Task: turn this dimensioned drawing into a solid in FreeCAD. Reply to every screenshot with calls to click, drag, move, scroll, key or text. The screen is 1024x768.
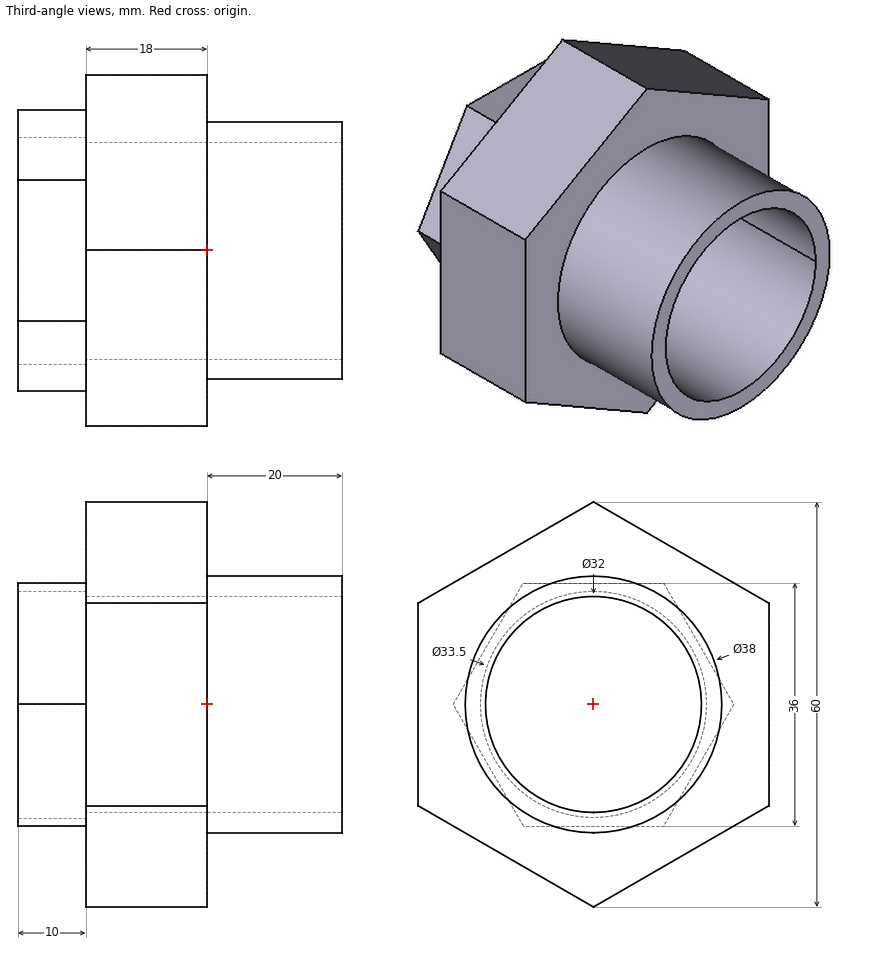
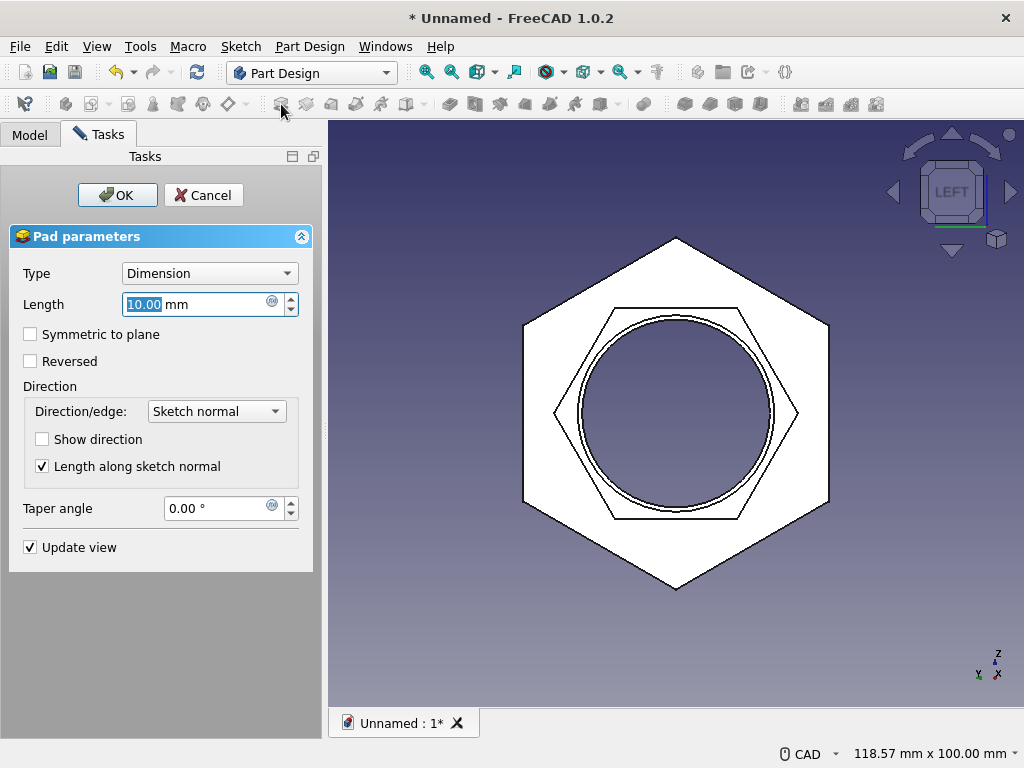
text(10)
key(Tab)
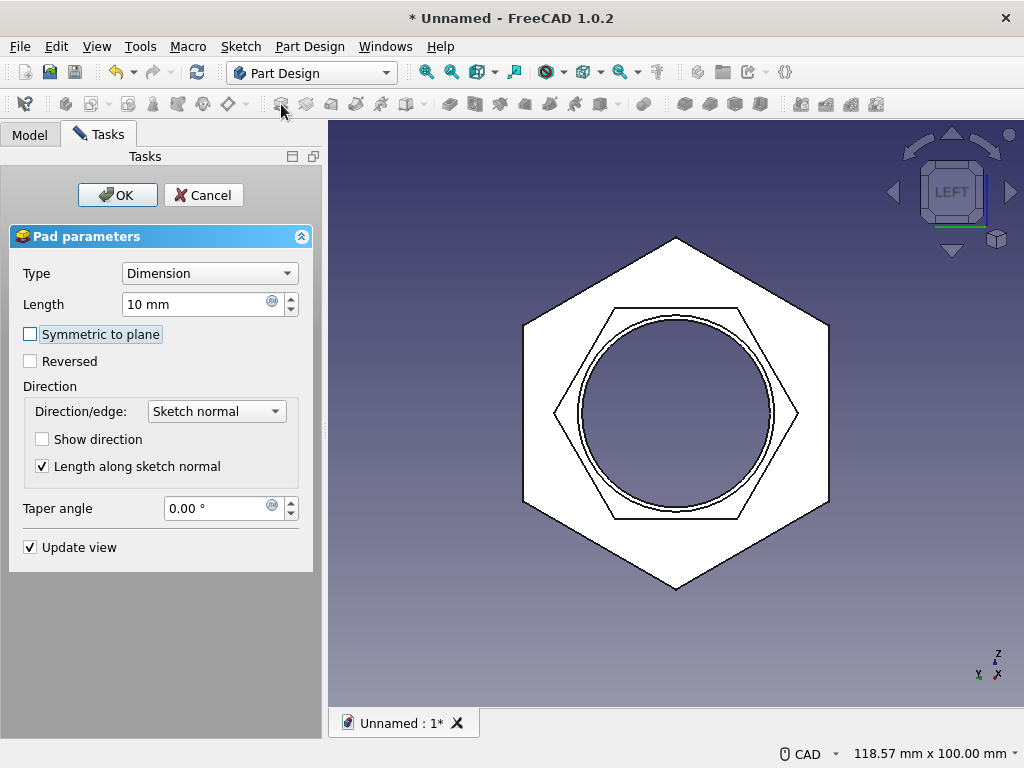
click(118, 195)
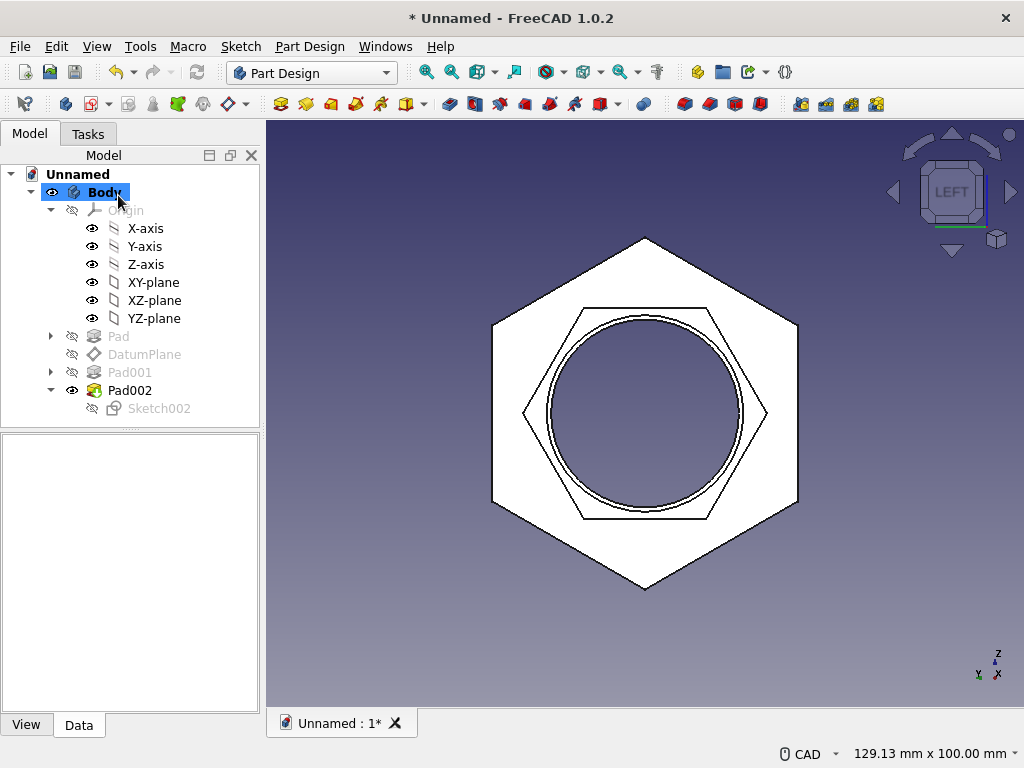
key(0)